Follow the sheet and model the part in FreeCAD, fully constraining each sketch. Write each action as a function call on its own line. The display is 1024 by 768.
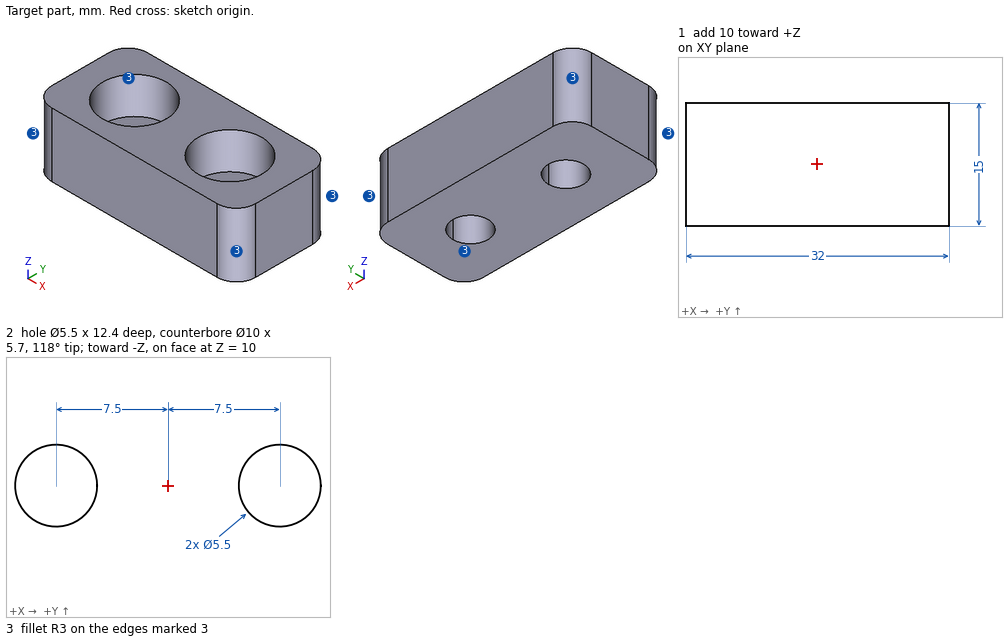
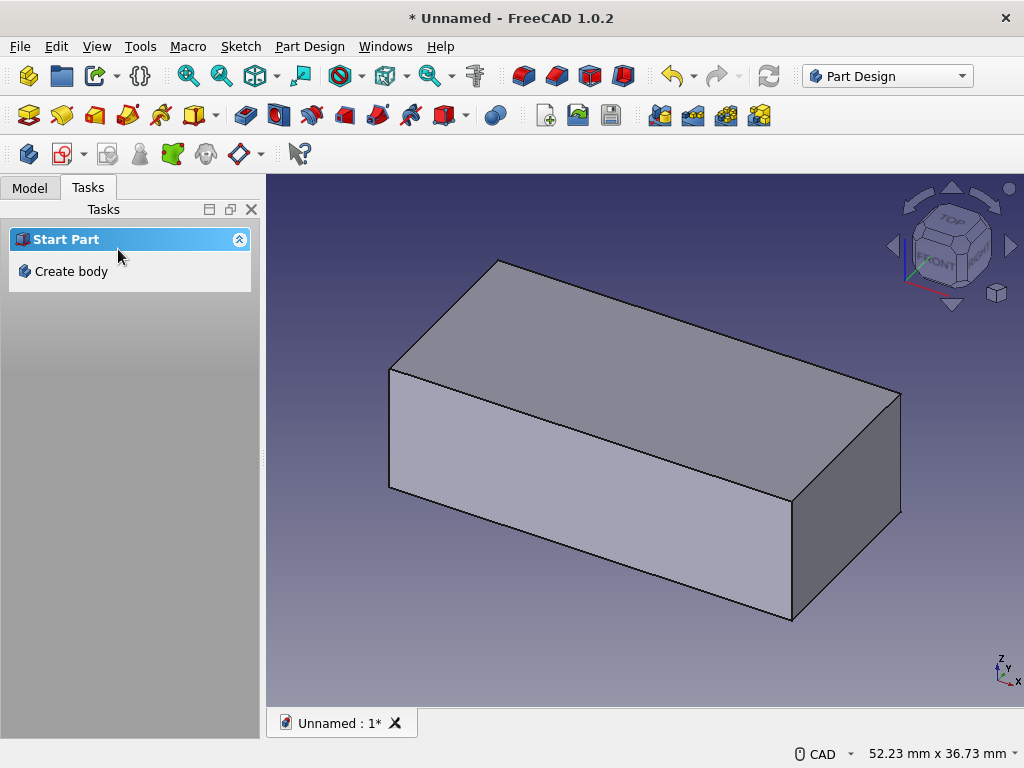
click(702, 399)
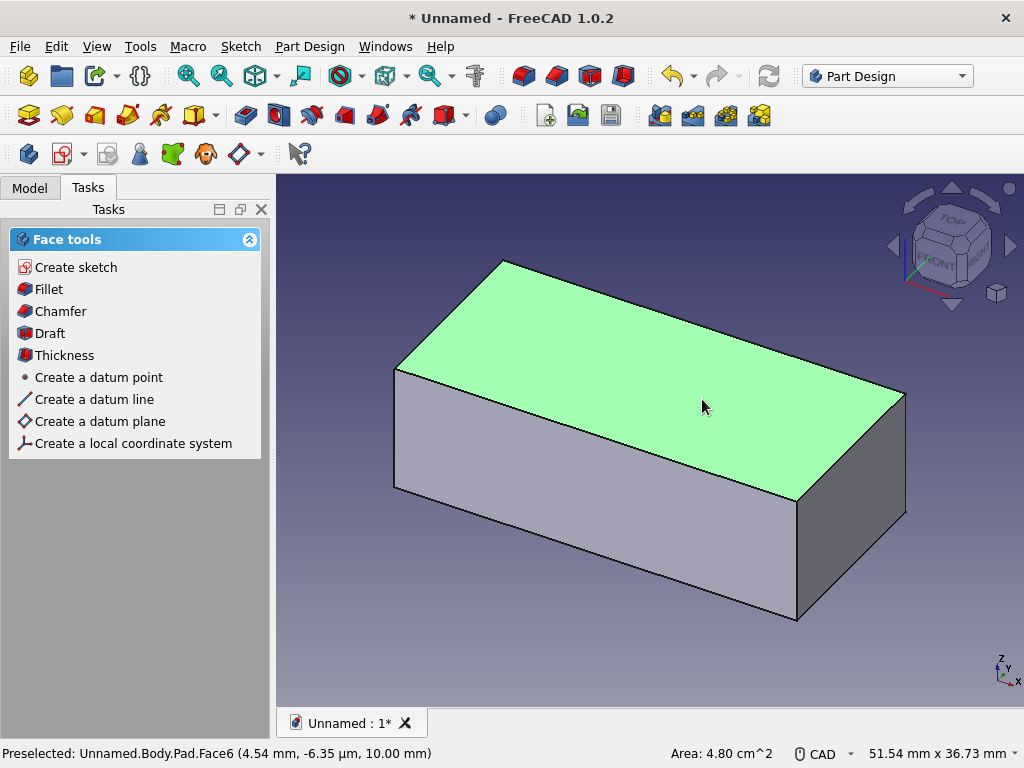
click(62, 154)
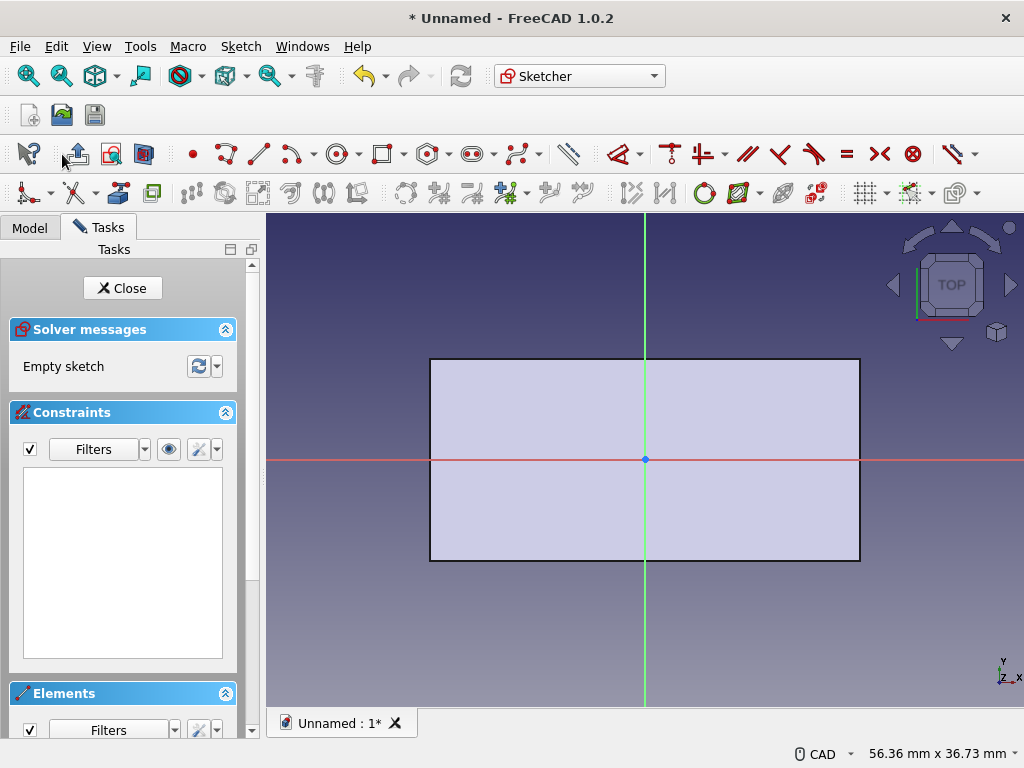
scroll(784, 460, up, 2)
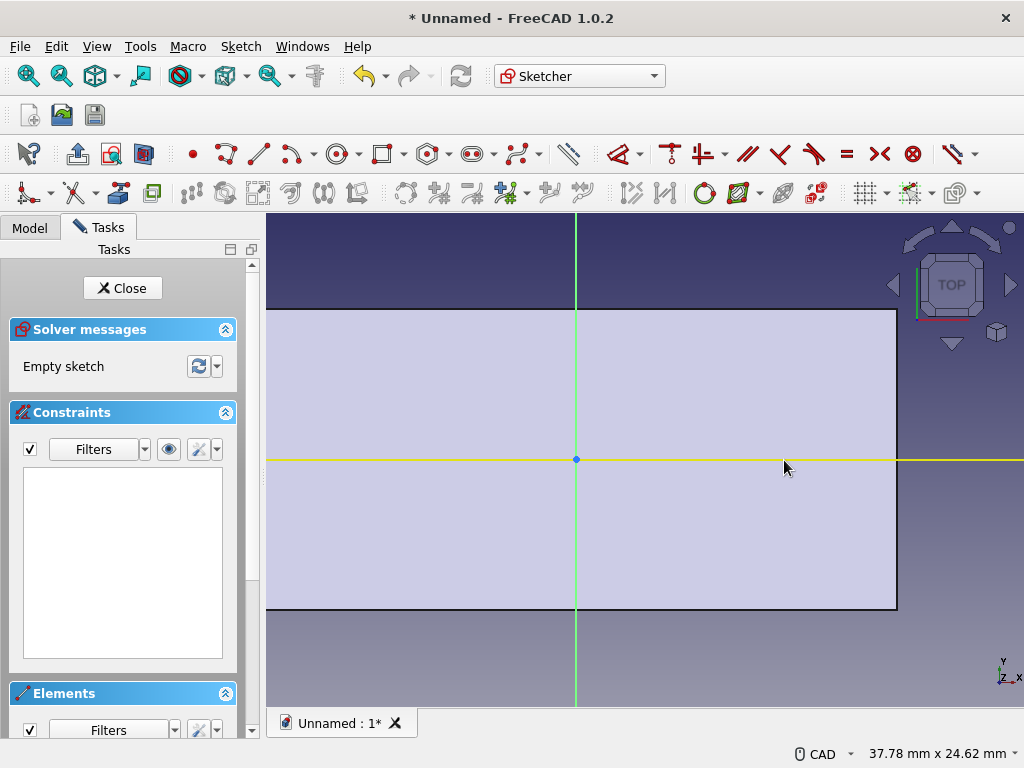
key(g)
key(c)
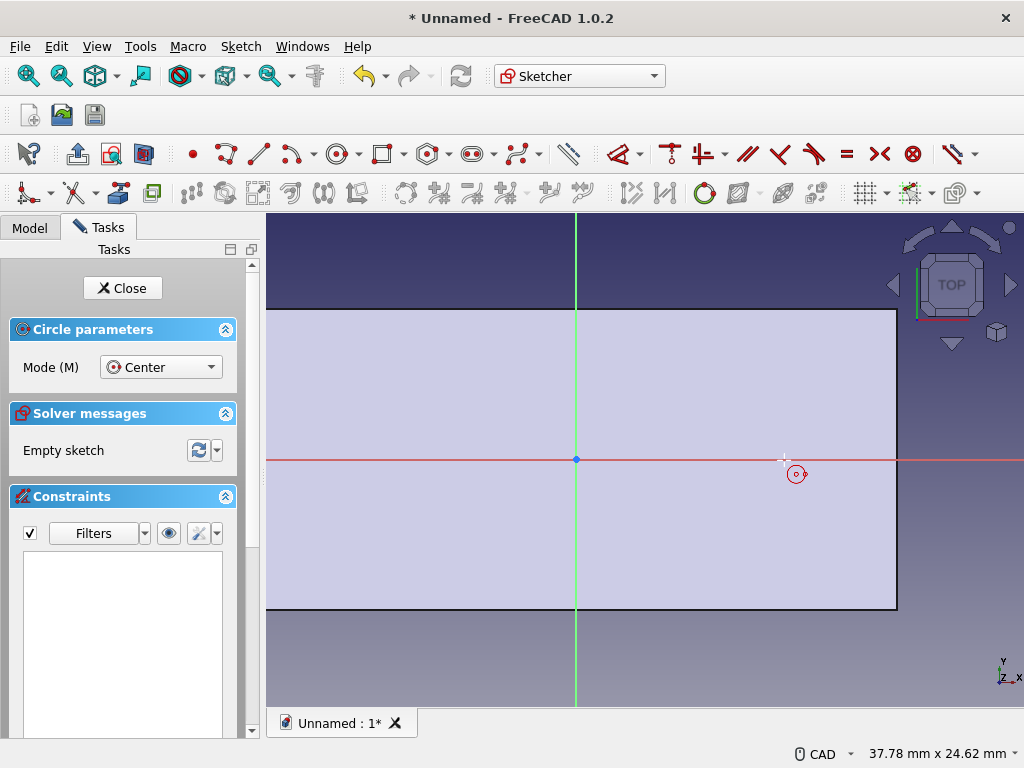
click(727, 460)
move(766, 421)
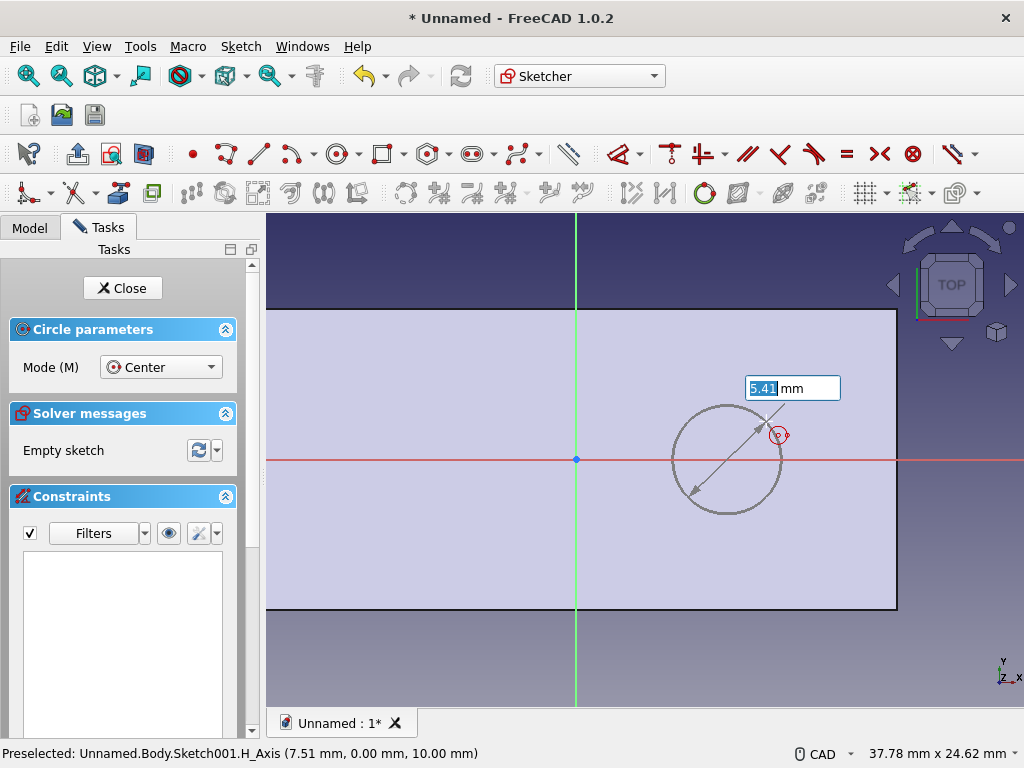
text(5.5)
key(Return)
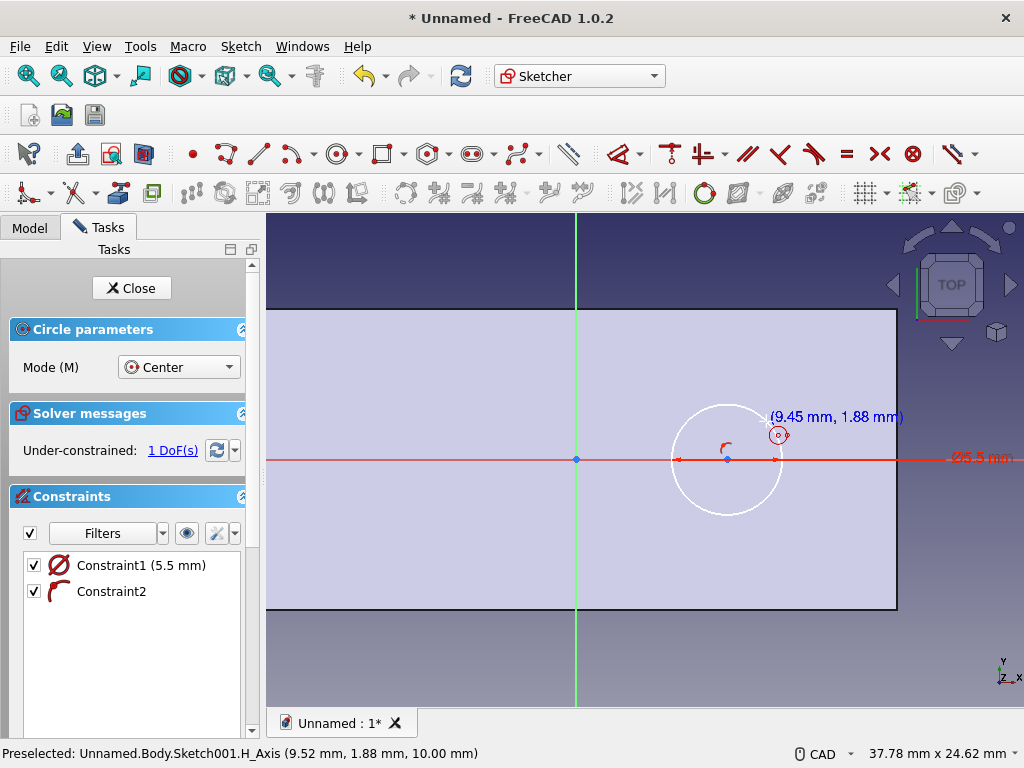
click(426, 460)
move(465, 421)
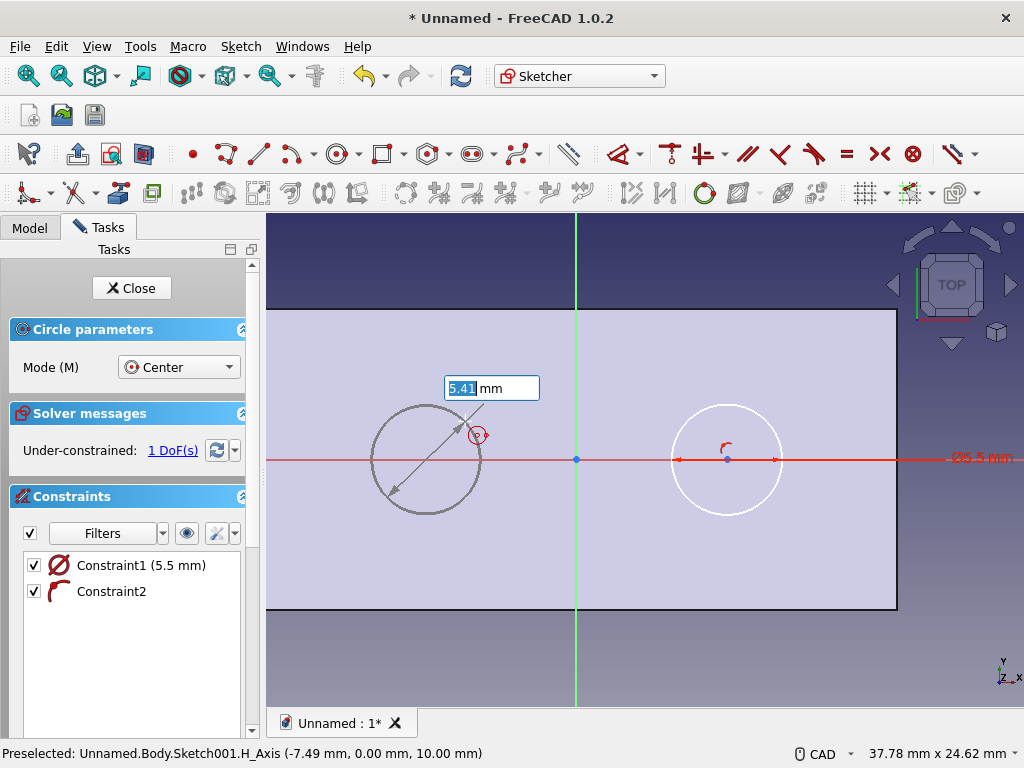
text(5.5)
key(Return)
key(Escape)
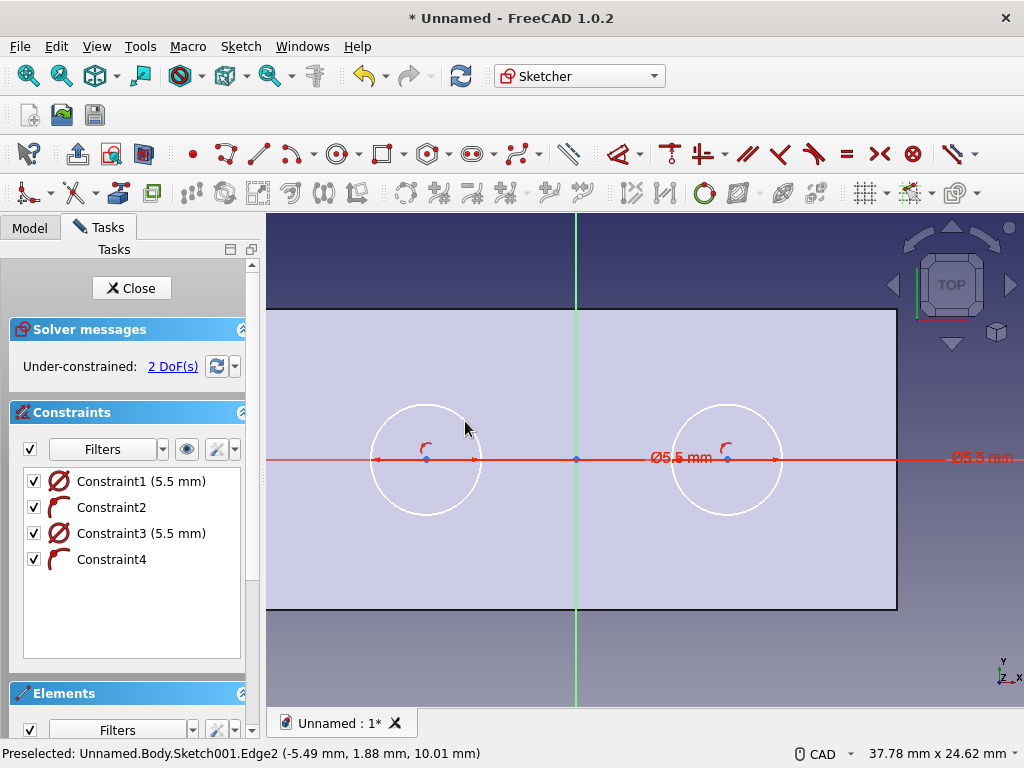
key(d)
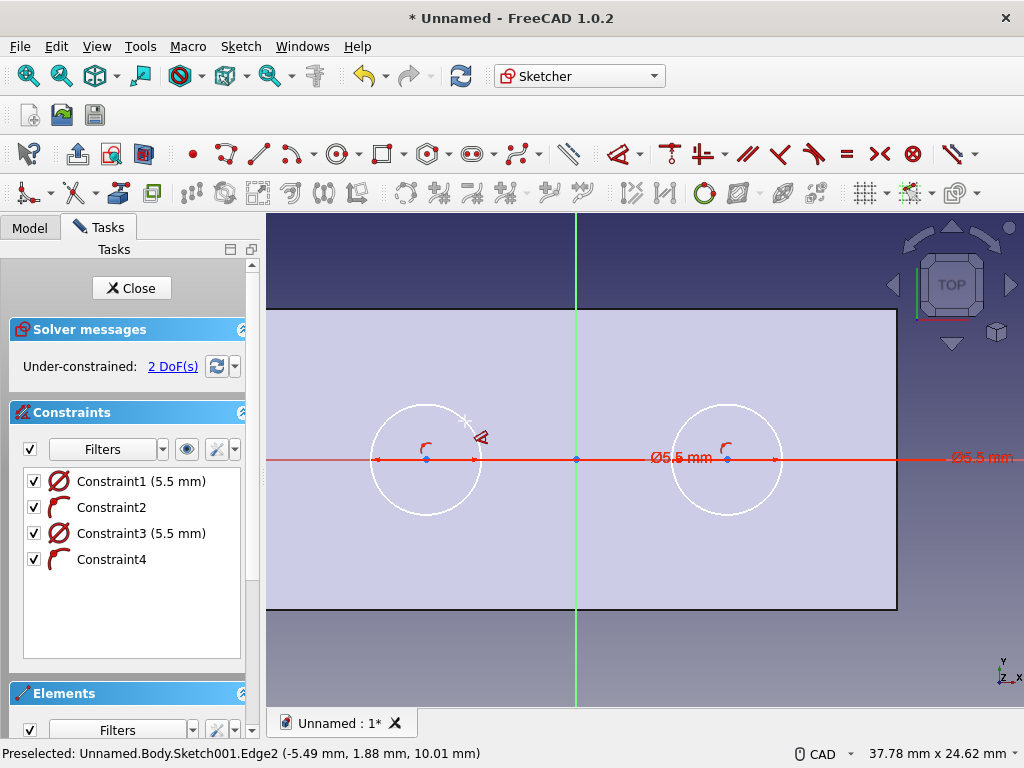
click(727, 460)
click(652, 494)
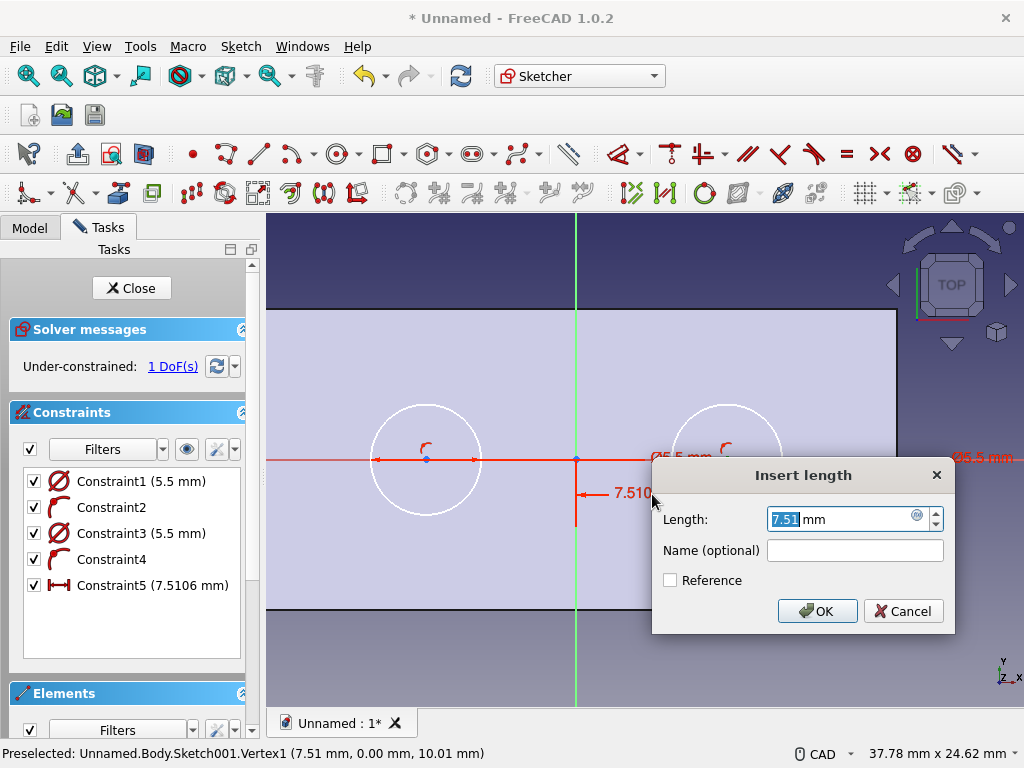
text(7.5)
key(Return)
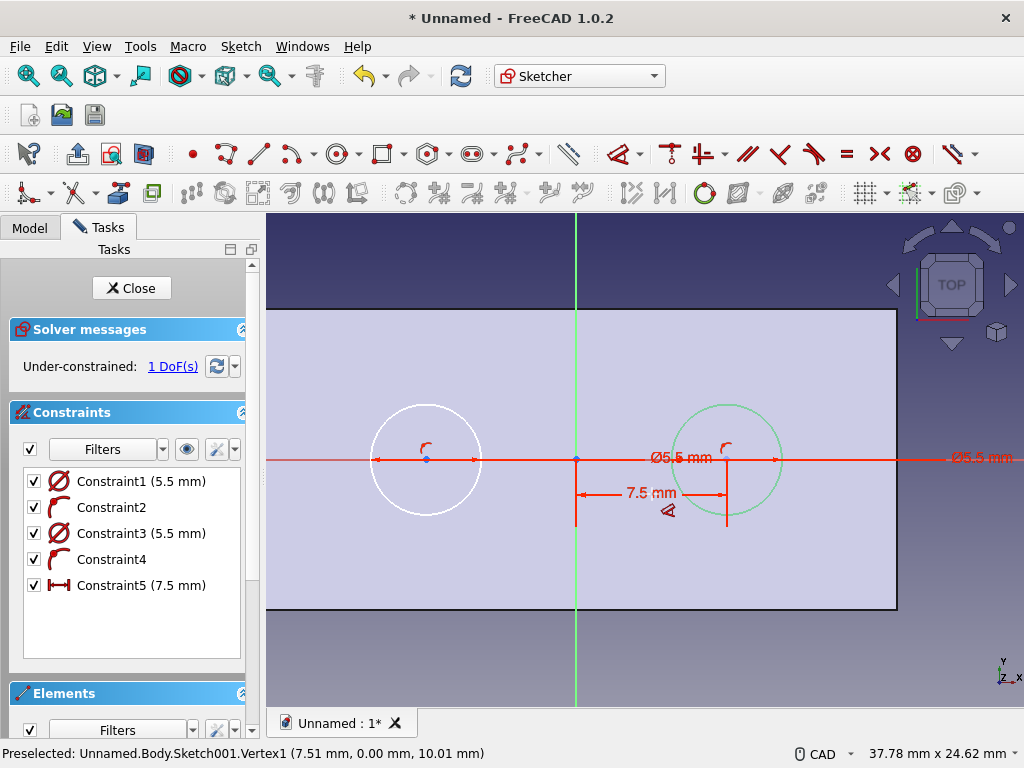
click(426, 460)
click(501, 494)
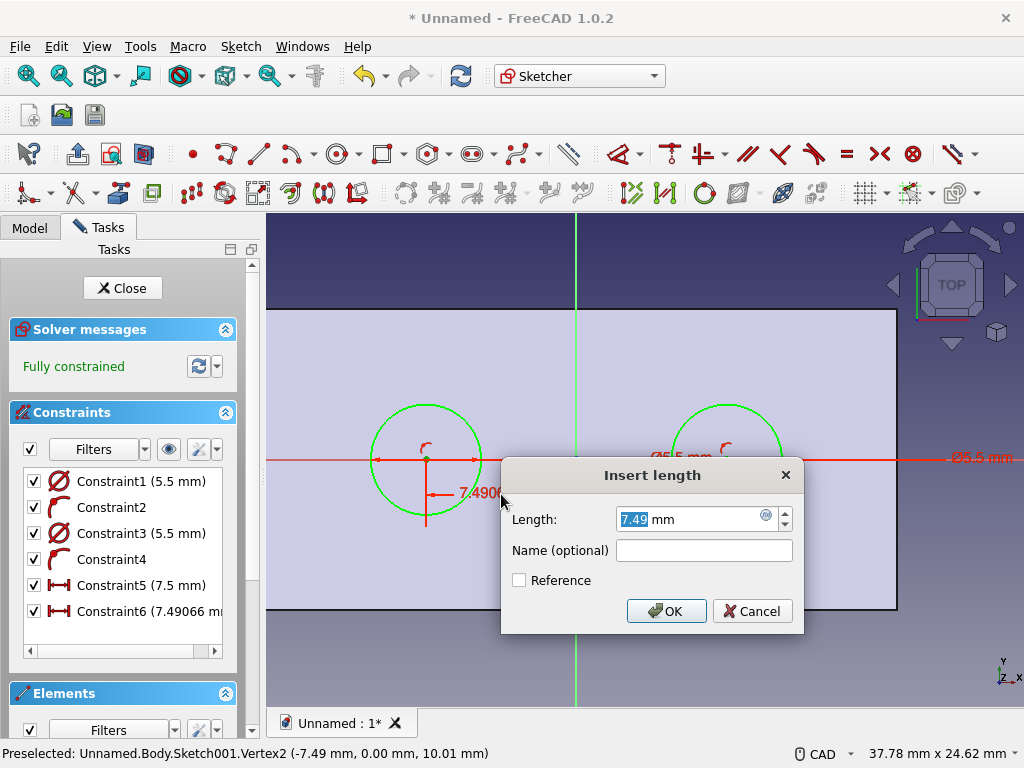
text(7.5)
key(Return)
key(Escape)